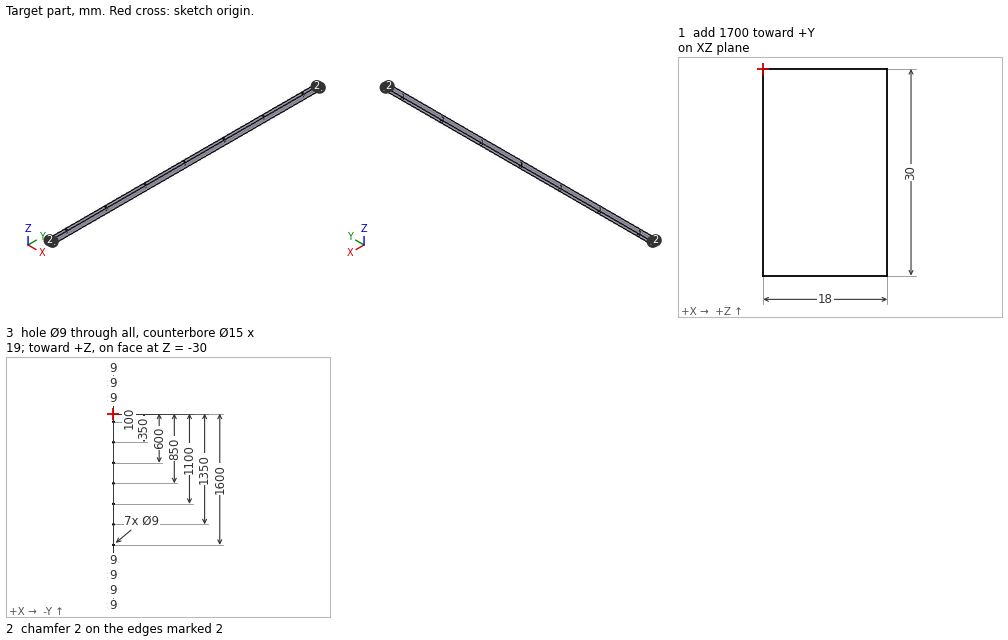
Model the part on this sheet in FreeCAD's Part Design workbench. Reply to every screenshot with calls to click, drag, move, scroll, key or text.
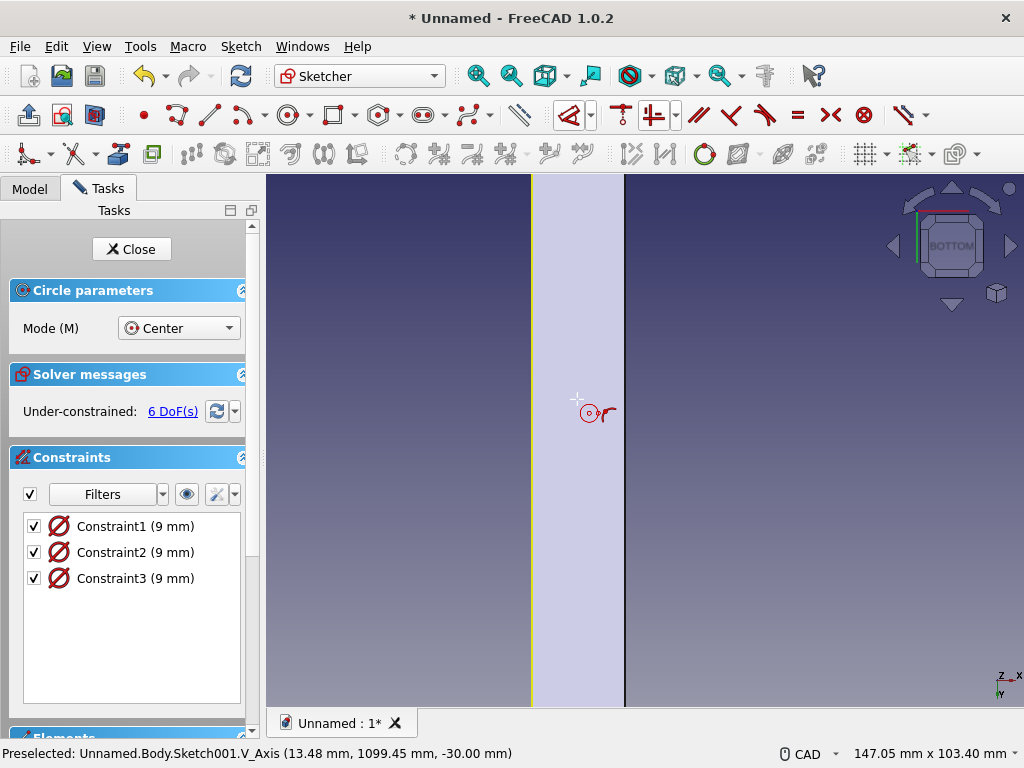
scroll(577, 389, down, 15)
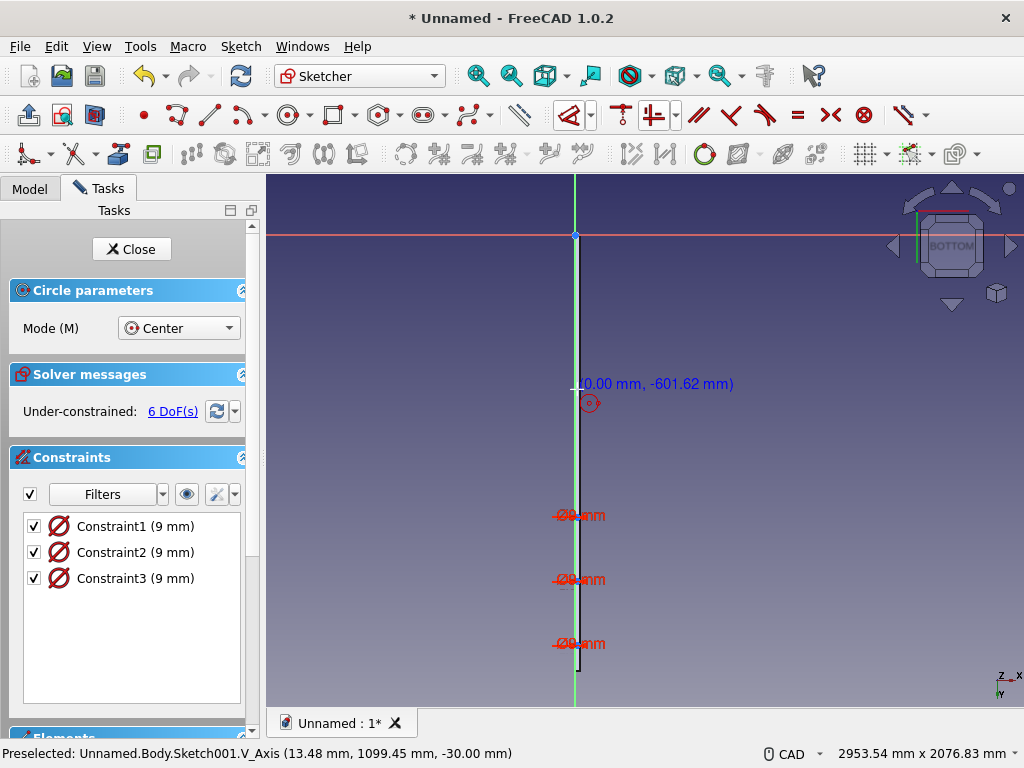
scroll(577, 389, up, 10)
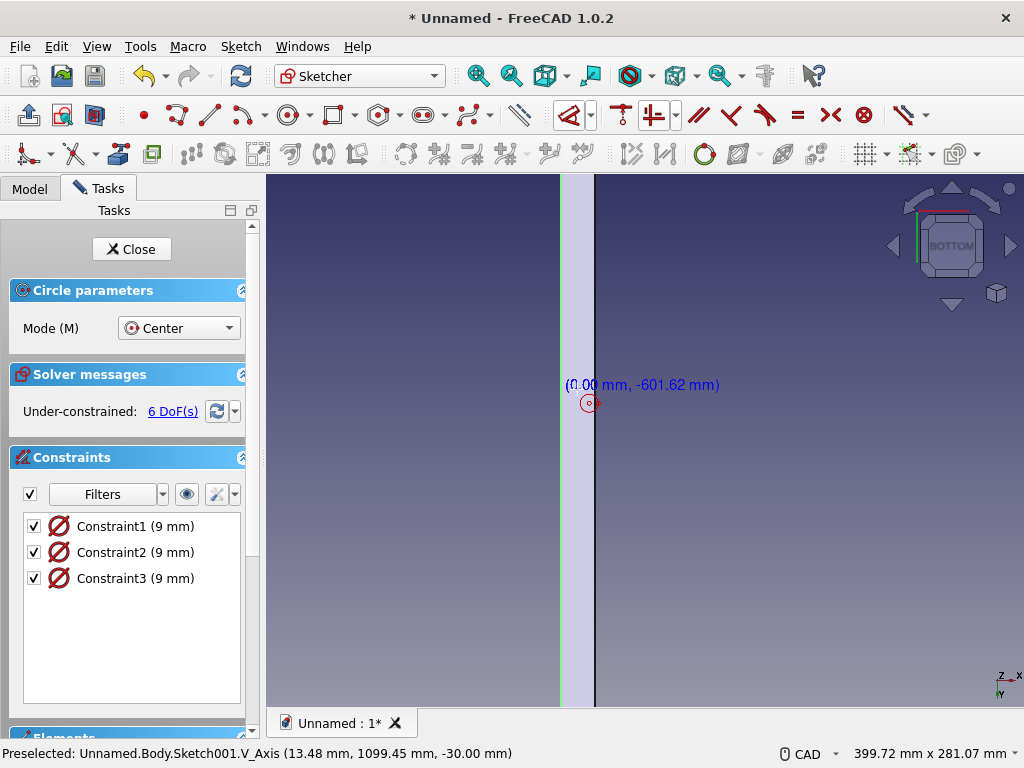
click(578, 387)
move(584, 381)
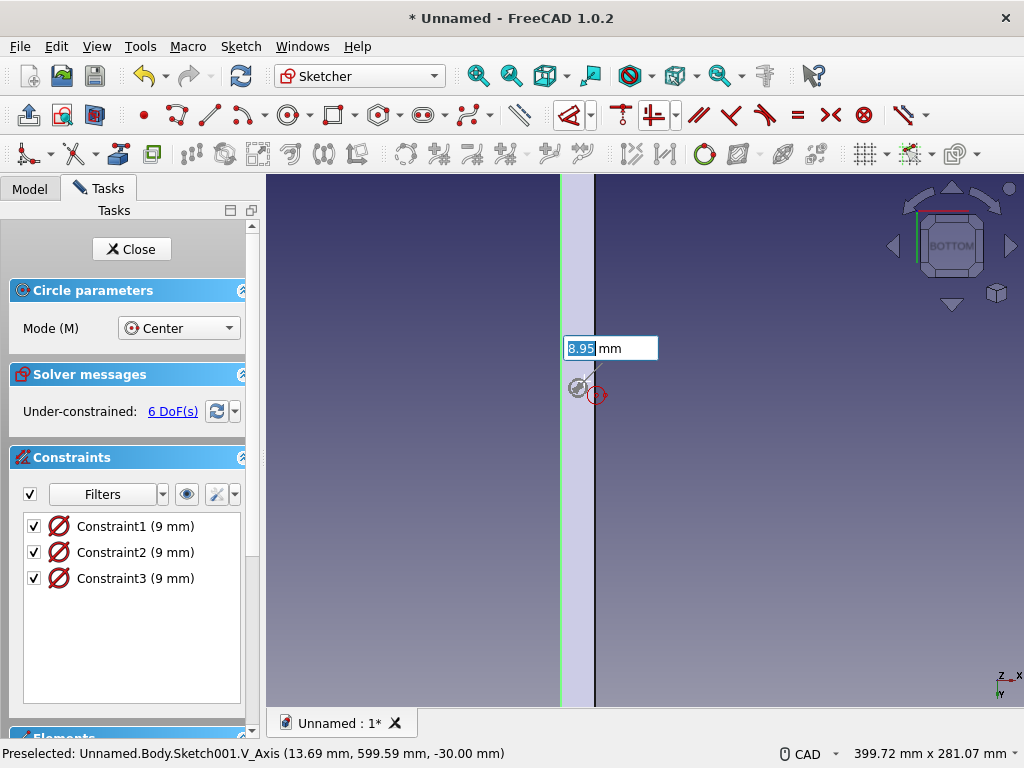
text(9)
key(Return)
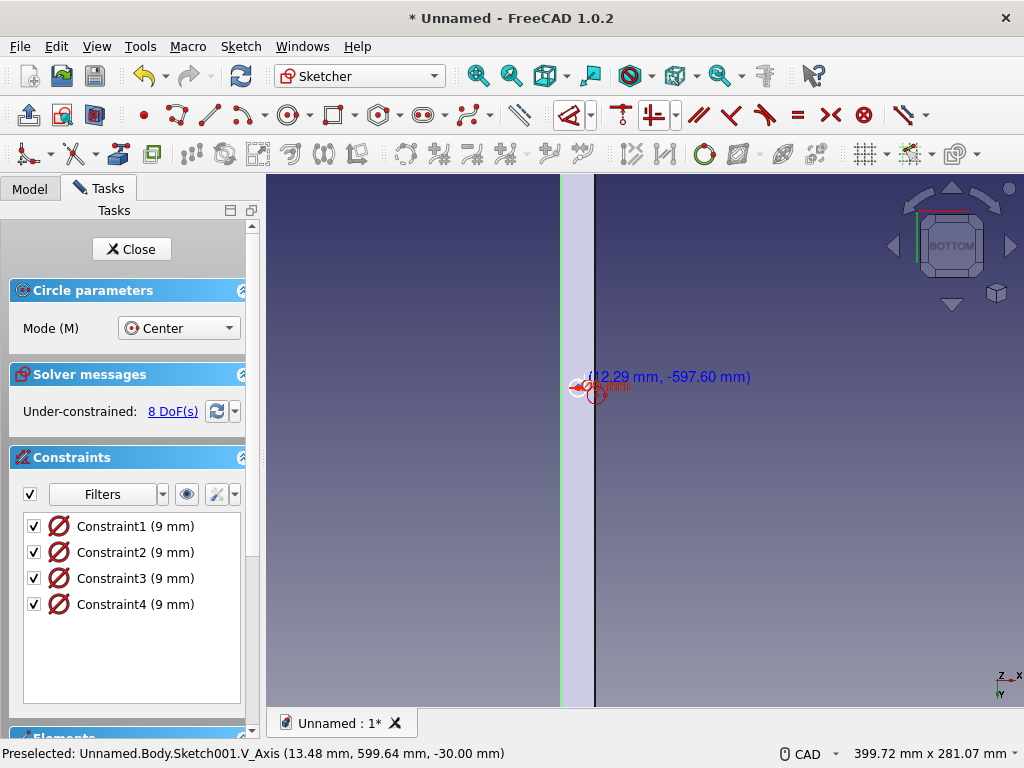
scroll(577, 399, down, 11)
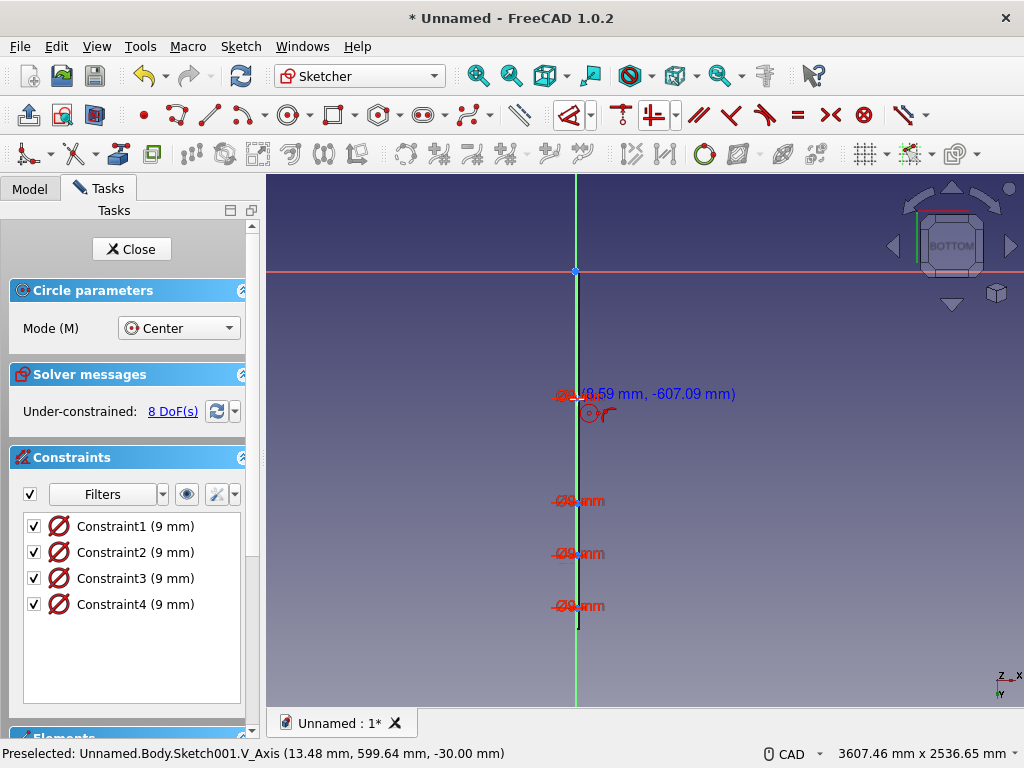
scroll(577, 345, up, 16)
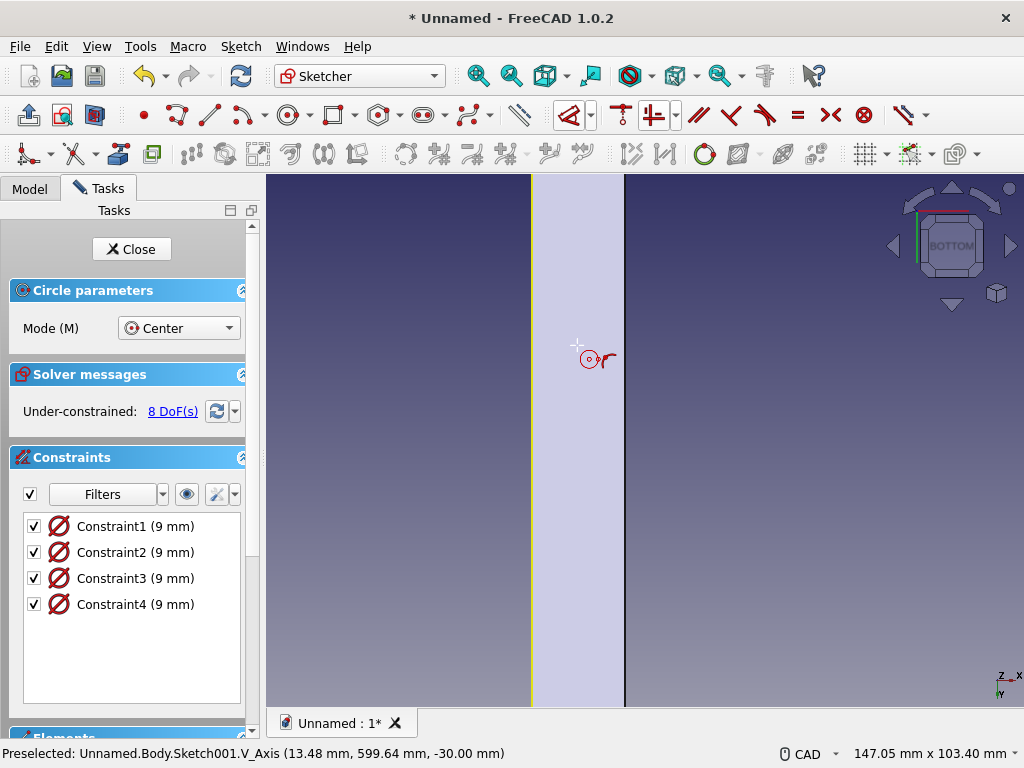
scroll(577, 323, down, 15)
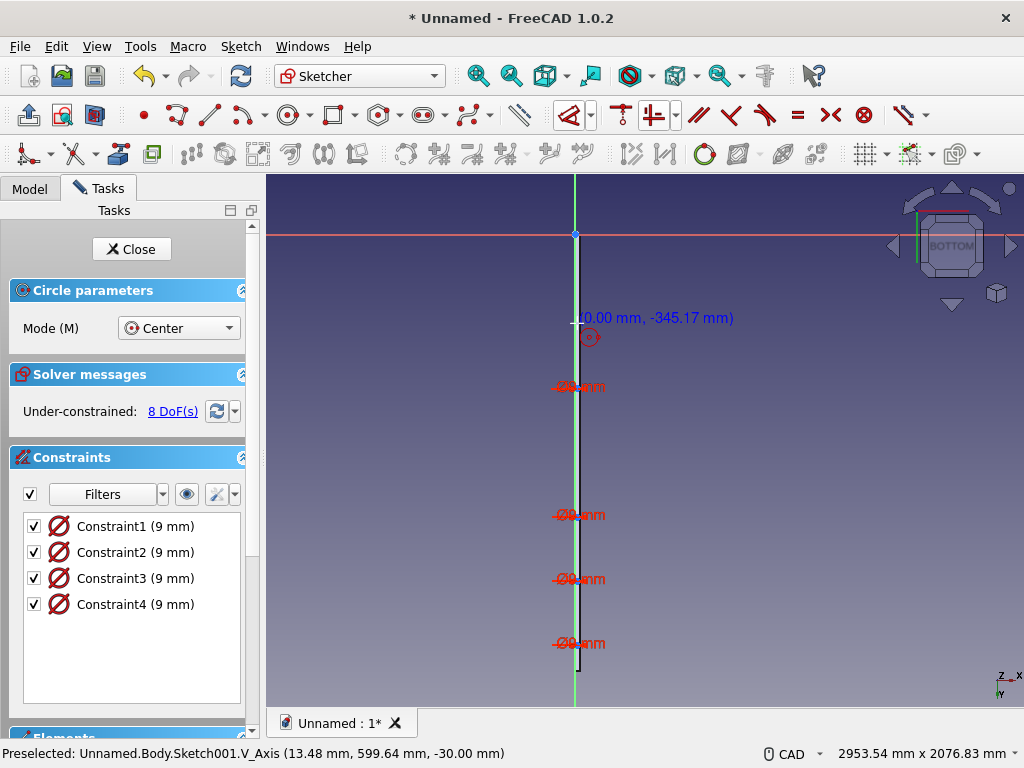
scroll(577, 325, up, 10)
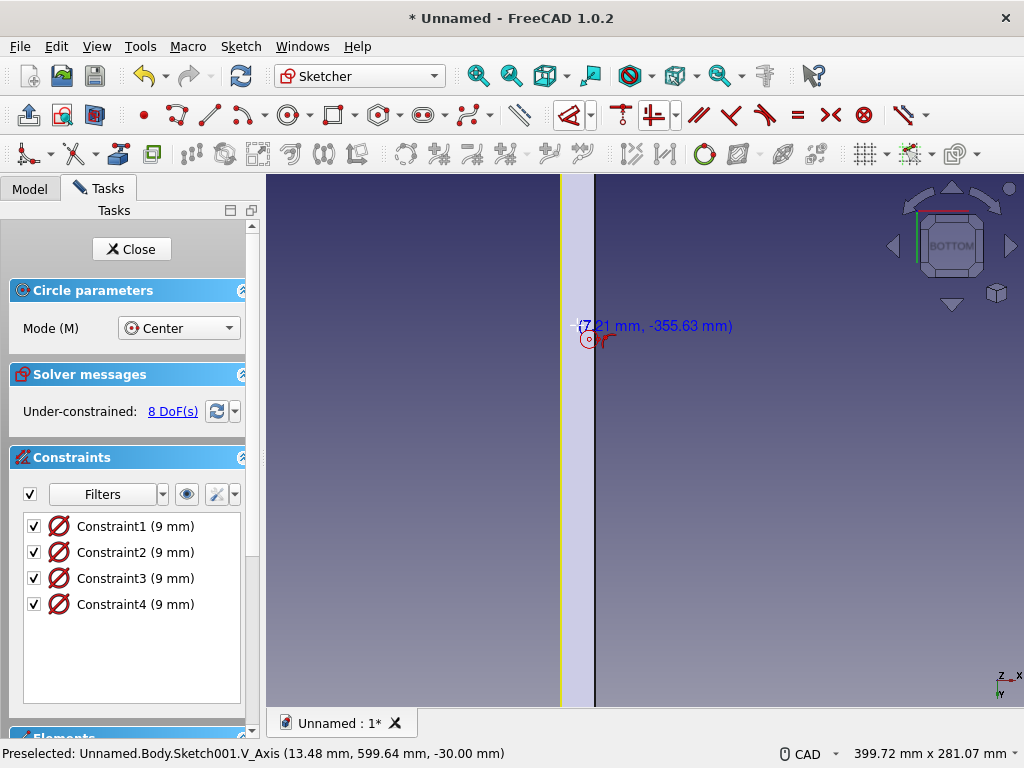
click(578, 320)
move(584, 314)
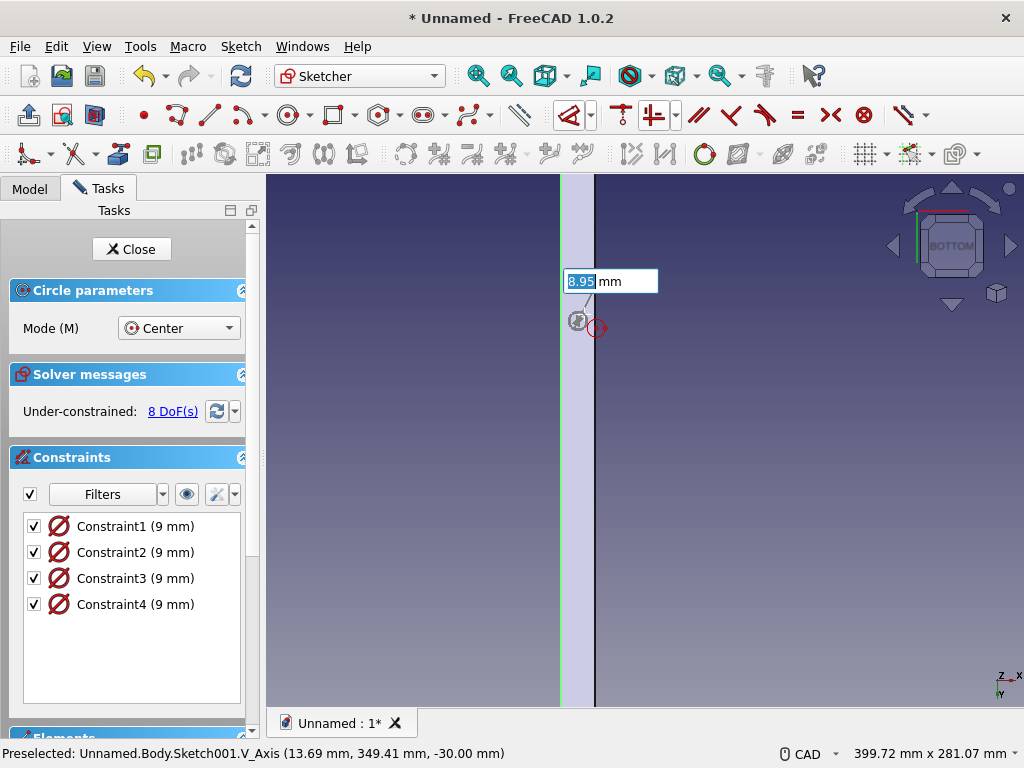
text(9)
key(Return)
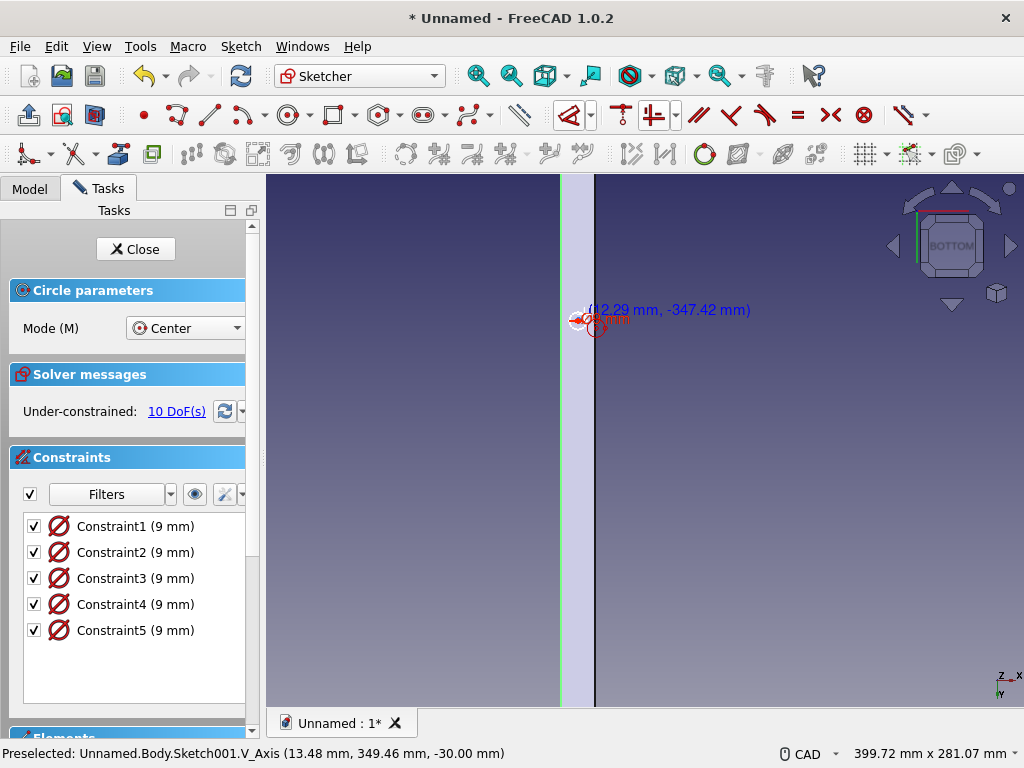
scroll(577, 349, down, 11)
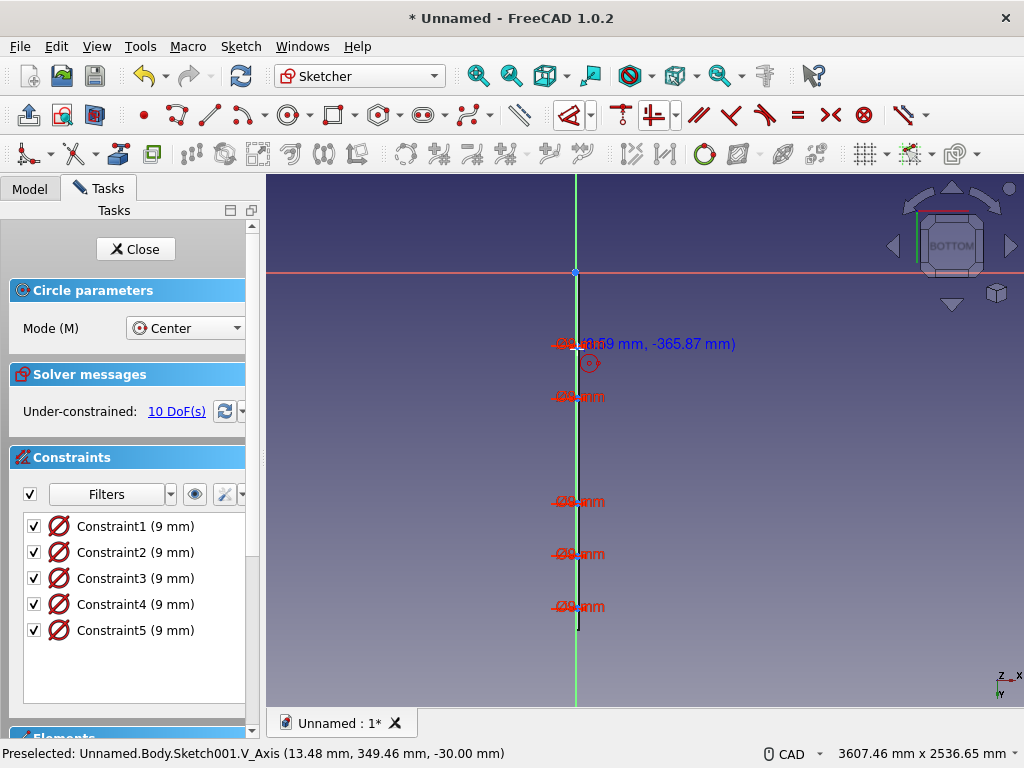
scroll(577, 294, up, 16)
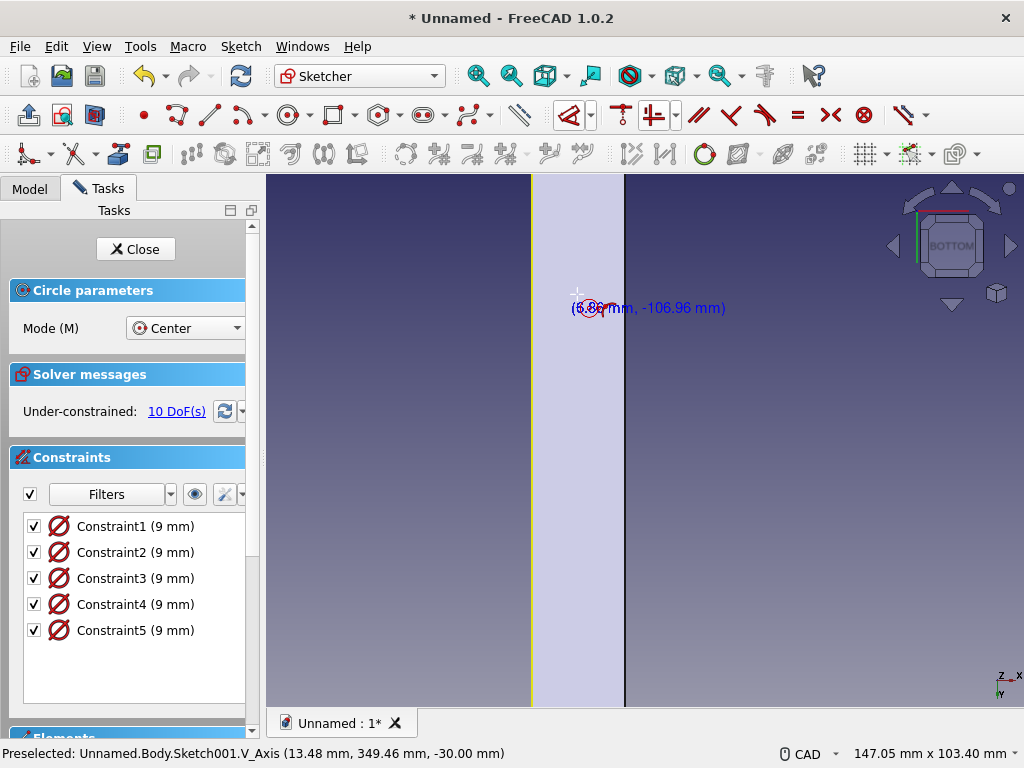
scroll(577, 259, down, 15)